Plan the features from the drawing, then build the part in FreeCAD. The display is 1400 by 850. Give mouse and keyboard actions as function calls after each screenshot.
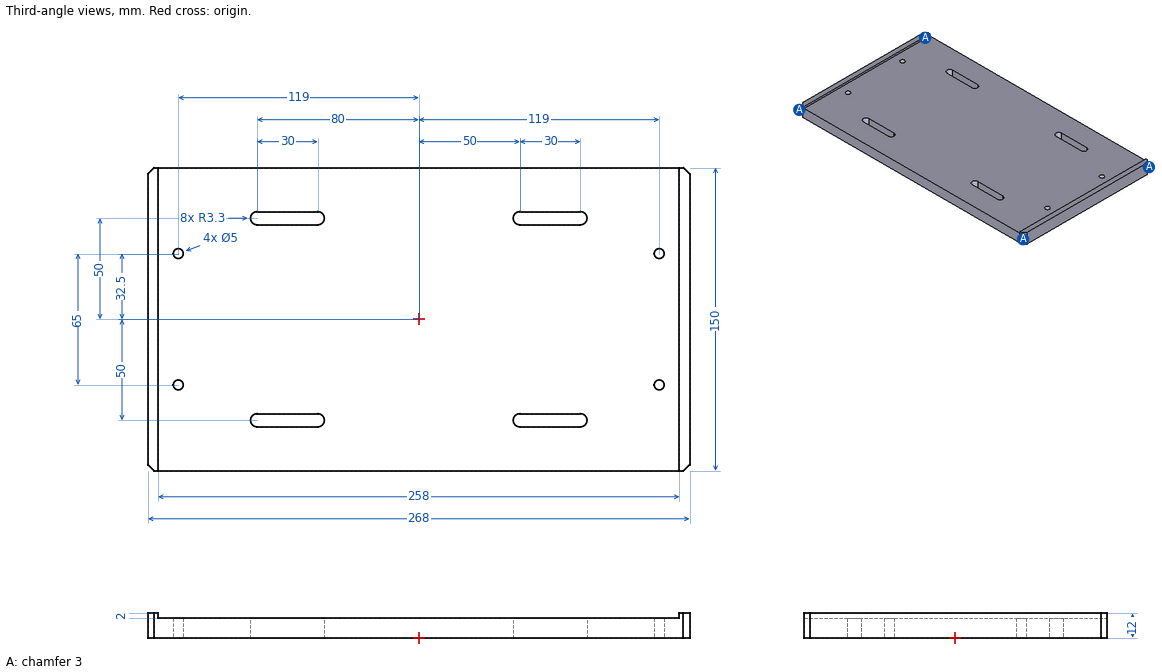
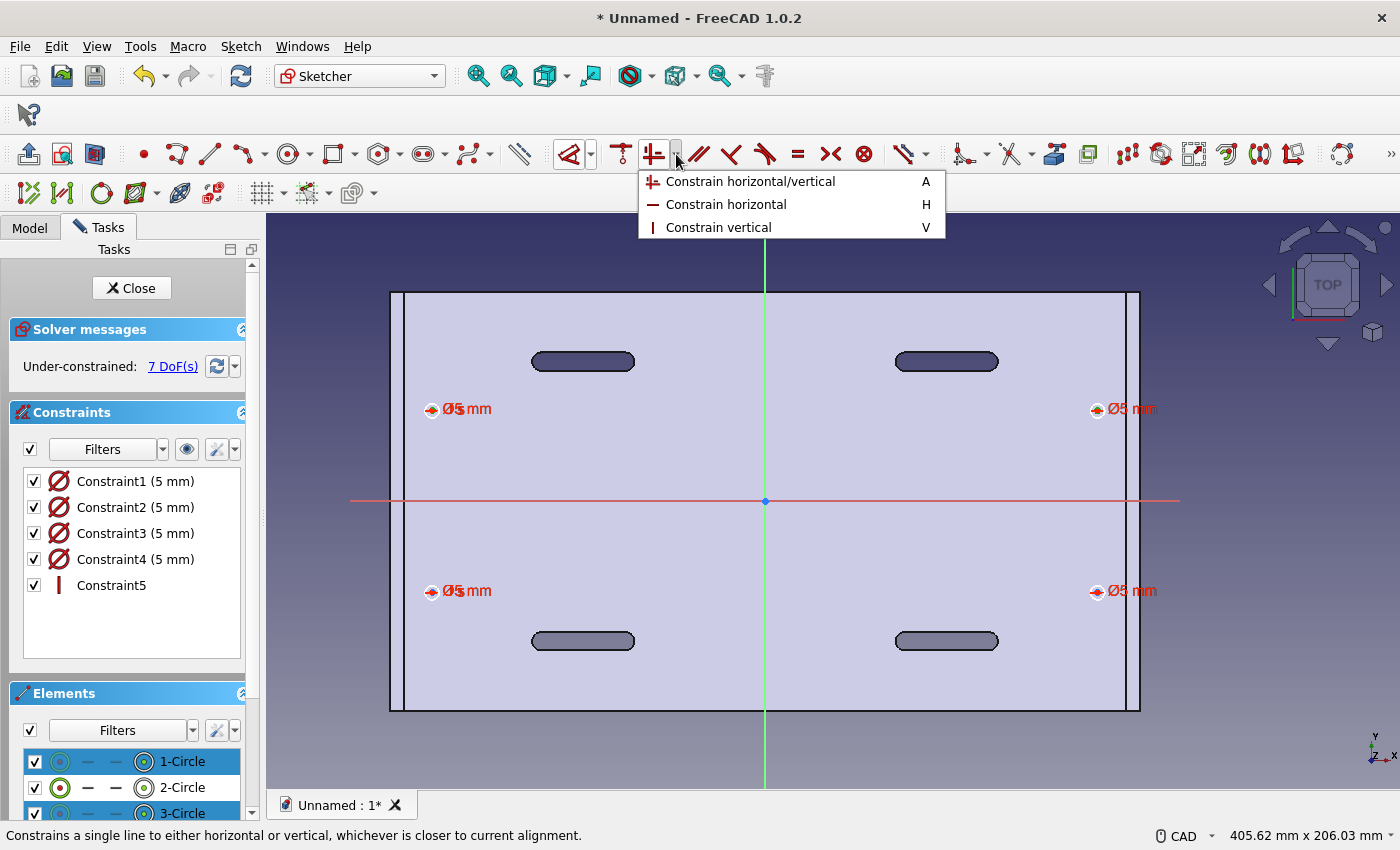
click(792, 204)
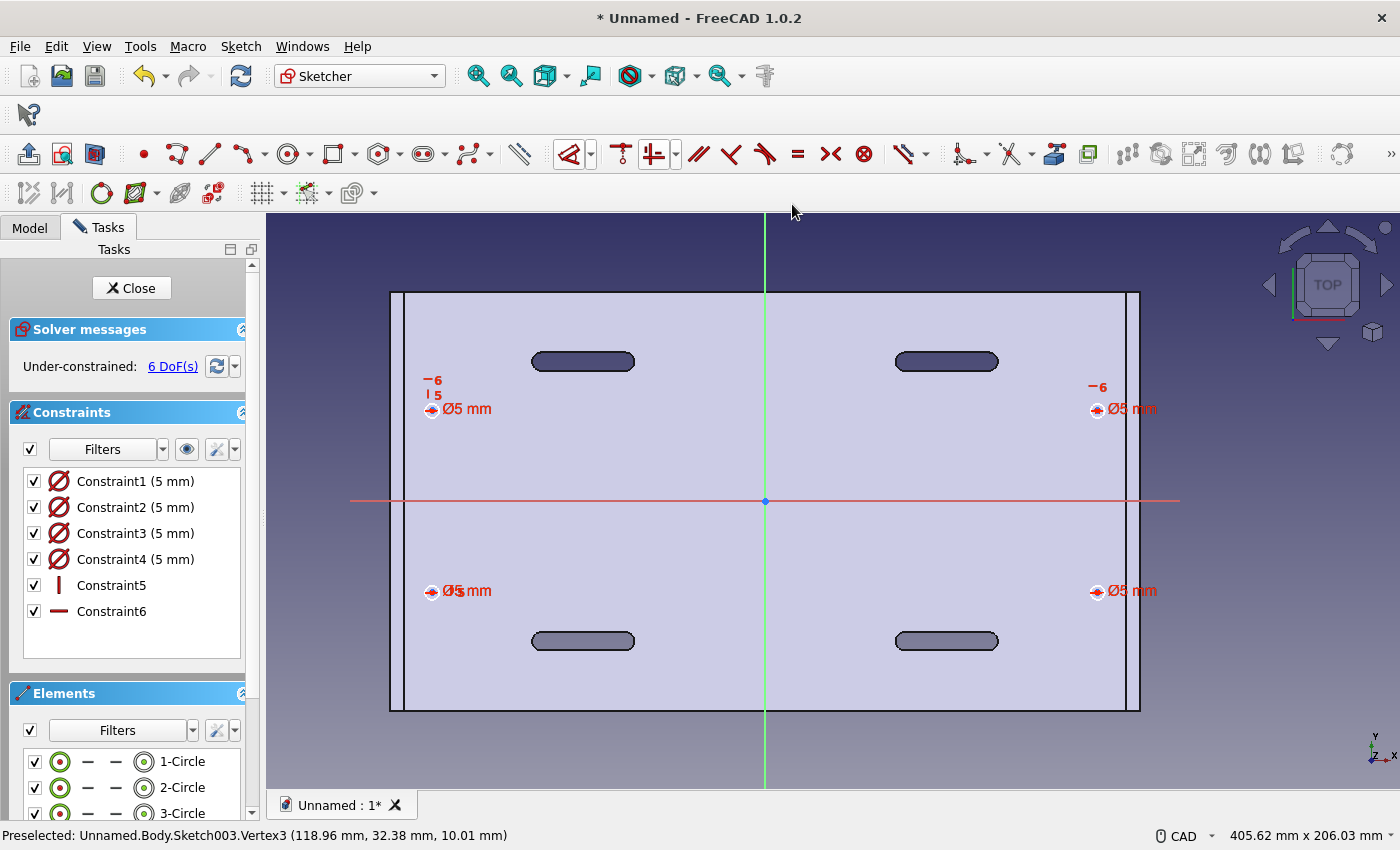
click(1098, 411)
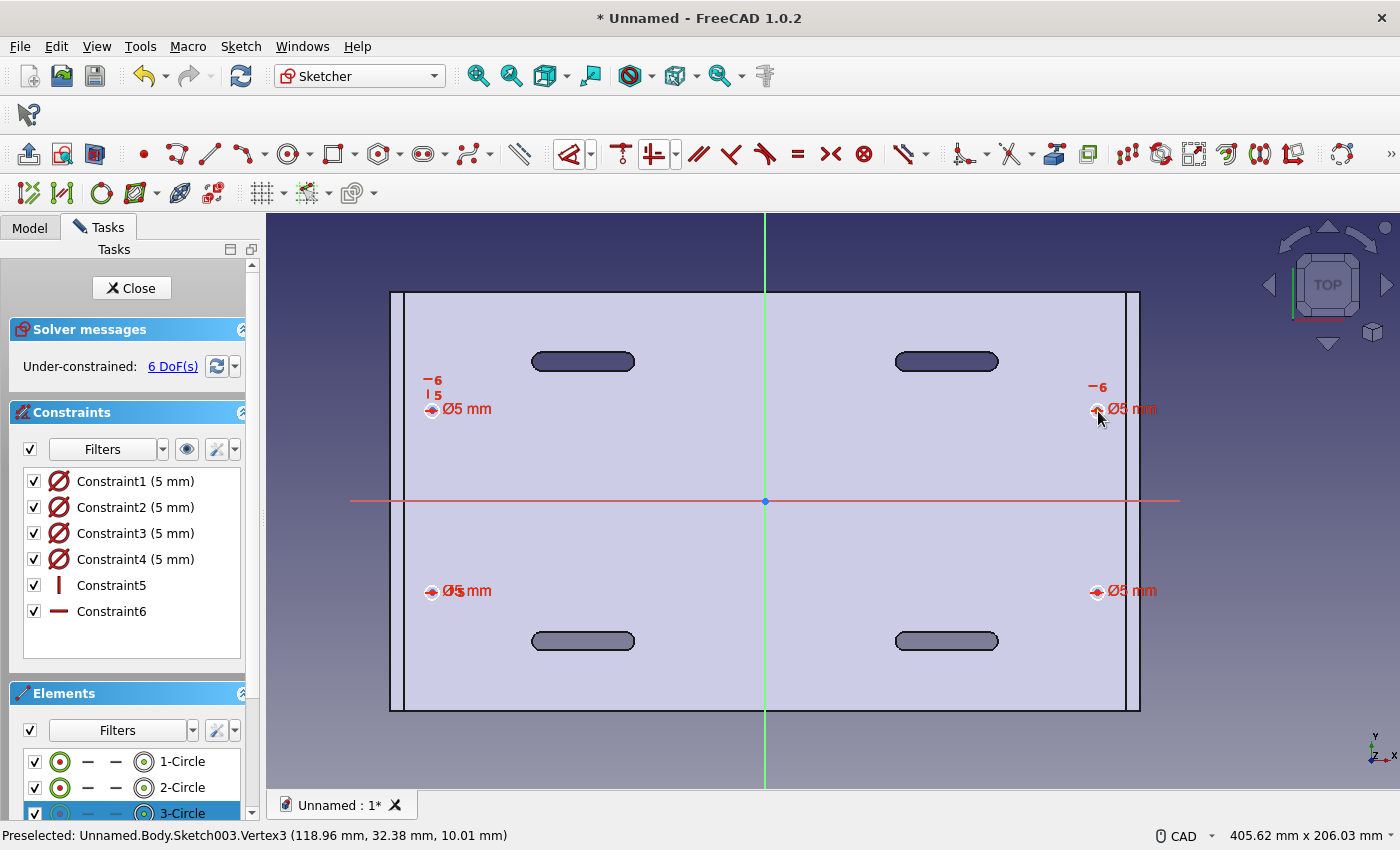
click(1098, 593)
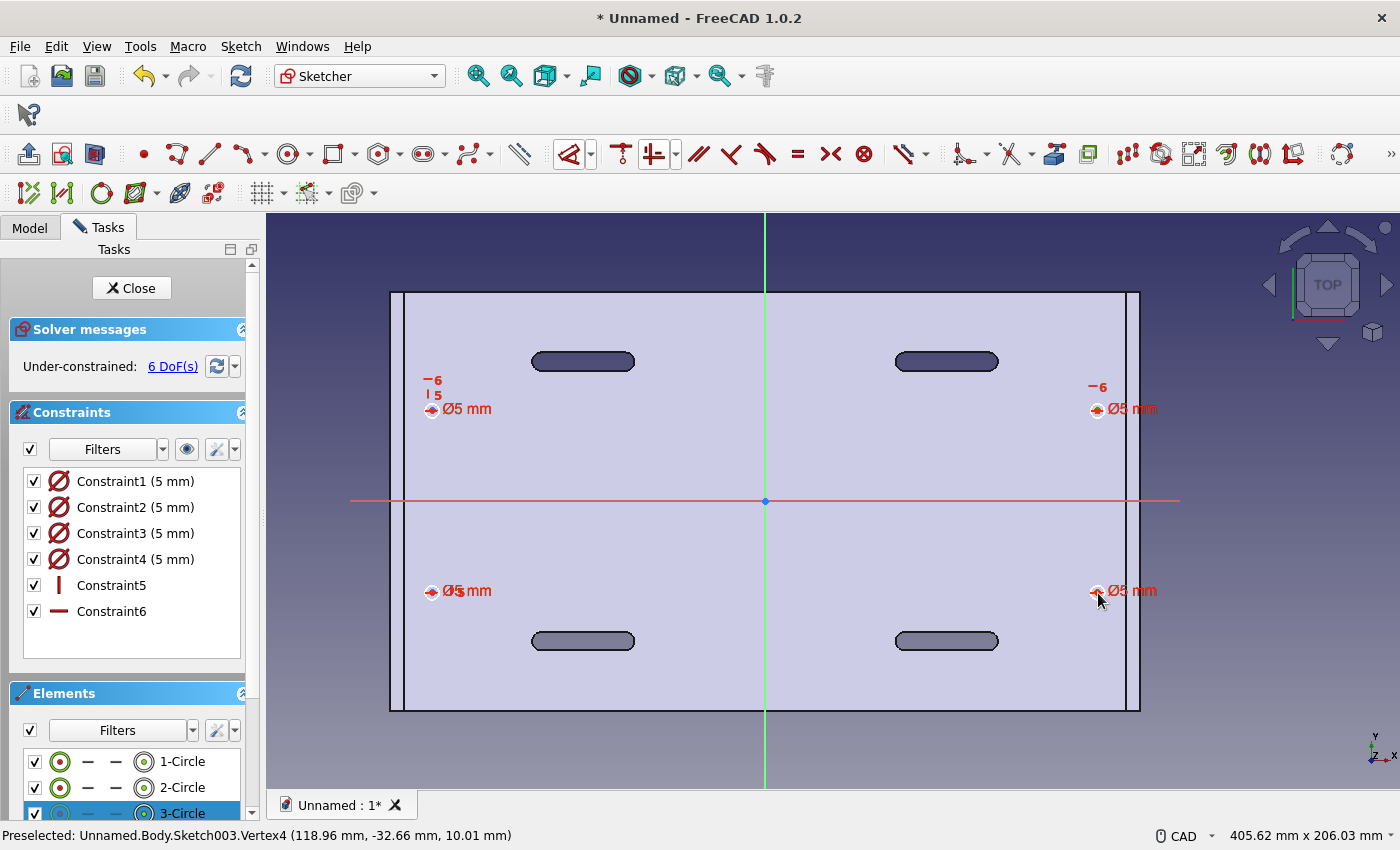
click(676, 154)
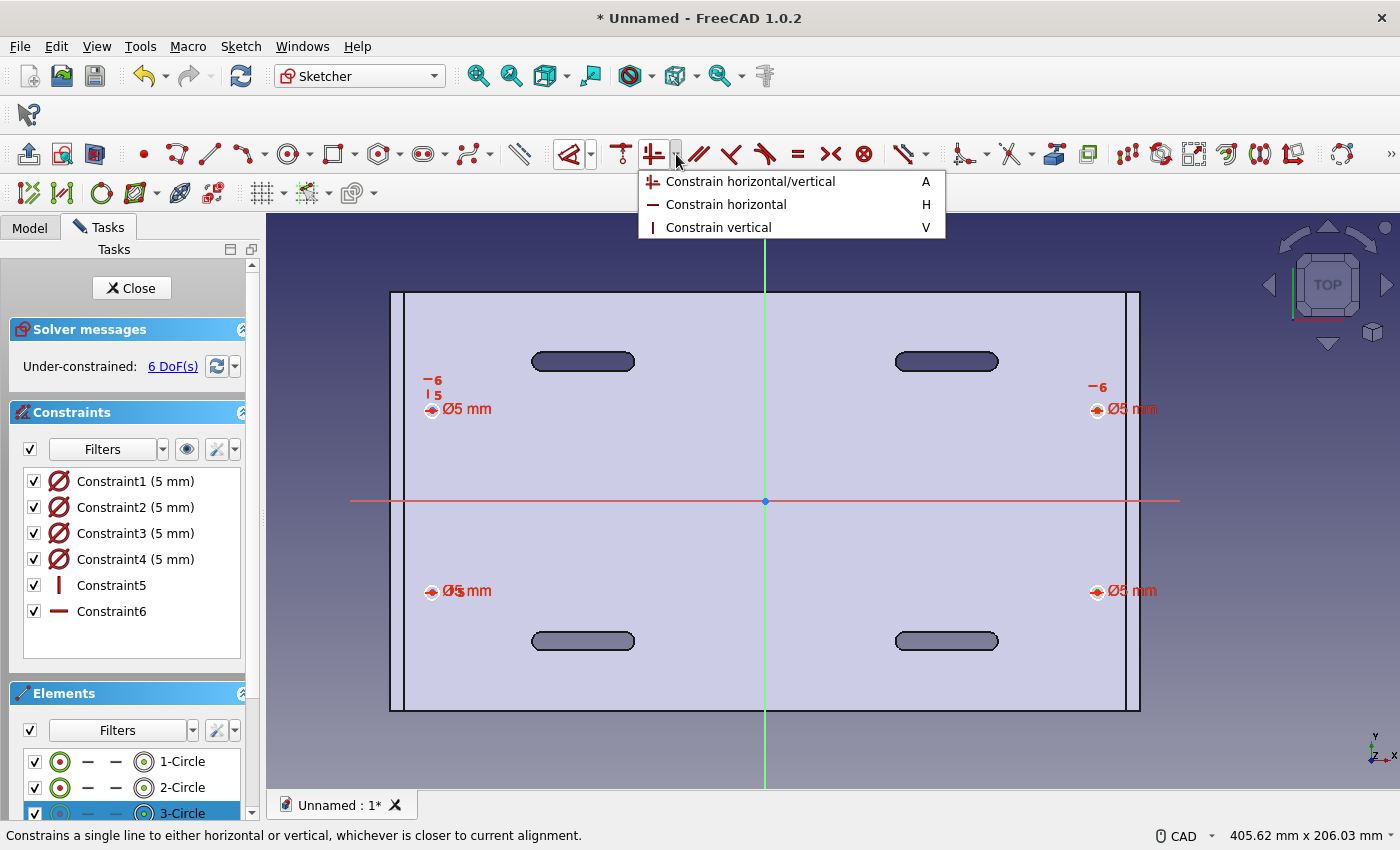
click(792, 228)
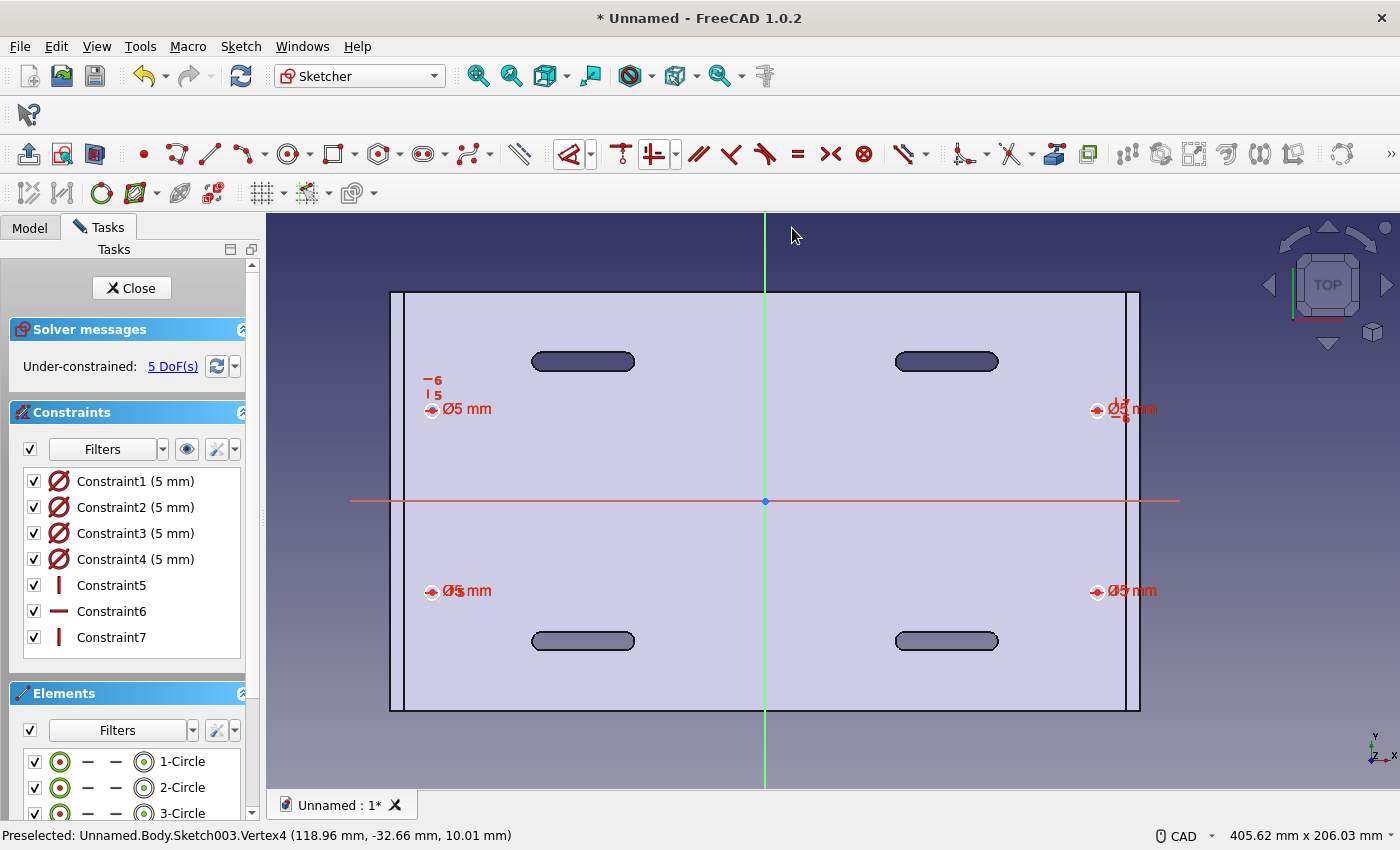
click(432, 593)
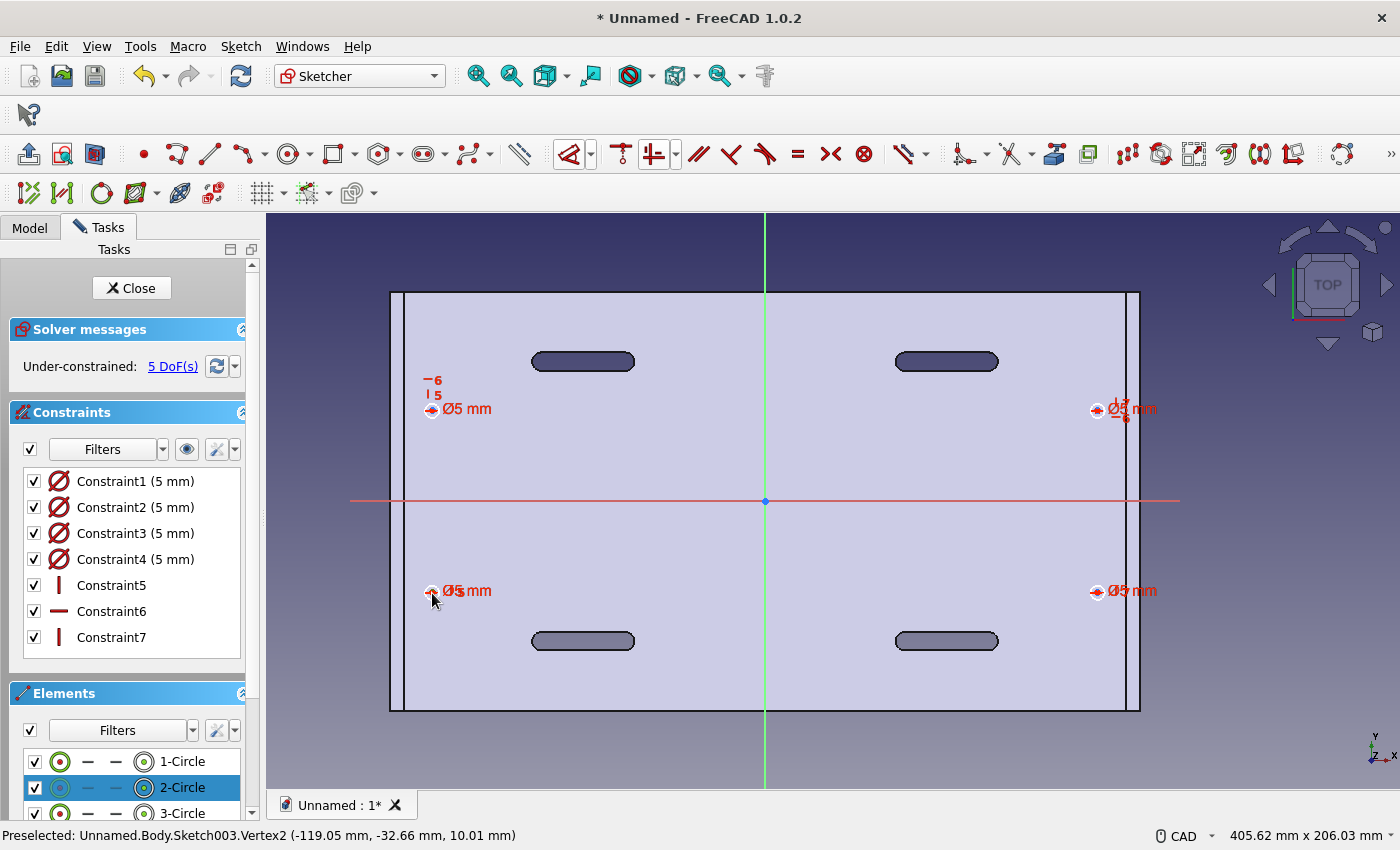
click(1098, 593)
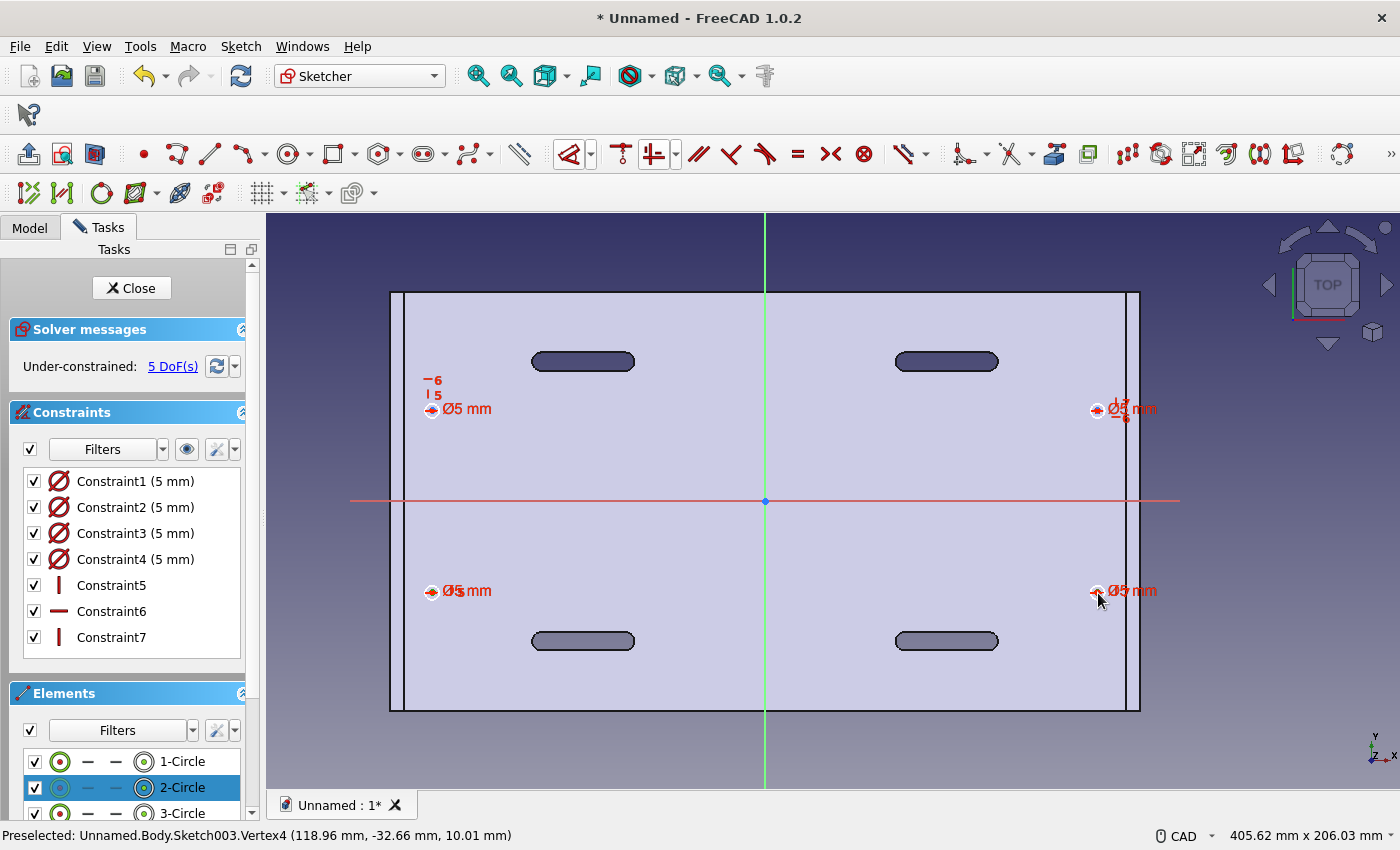
key(h)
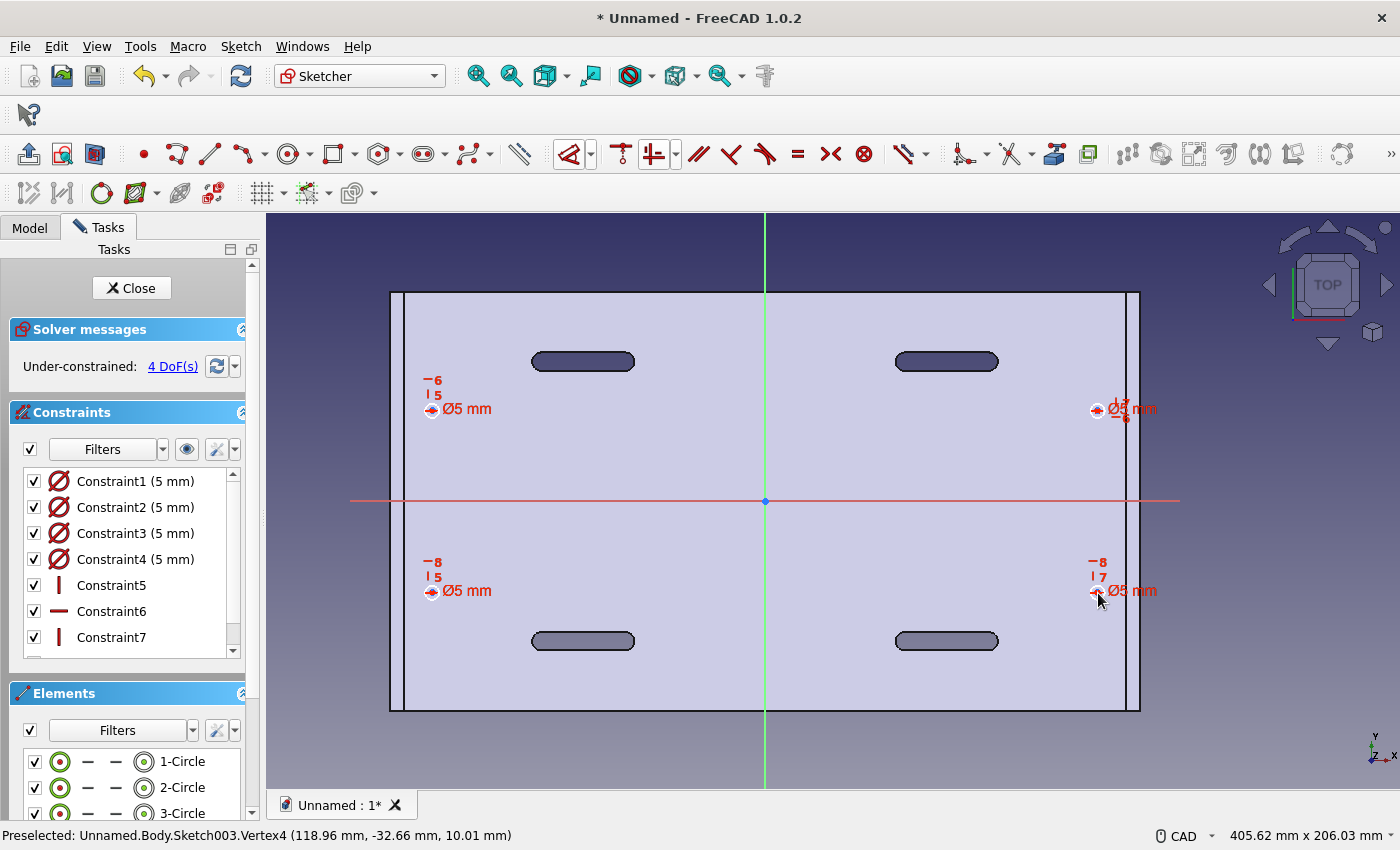
click(432, 411)